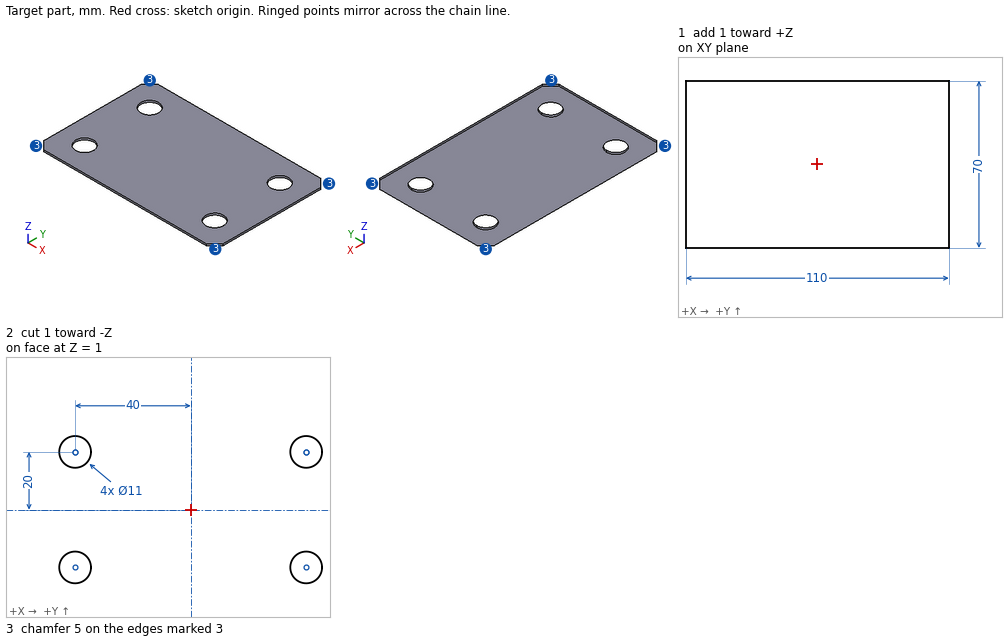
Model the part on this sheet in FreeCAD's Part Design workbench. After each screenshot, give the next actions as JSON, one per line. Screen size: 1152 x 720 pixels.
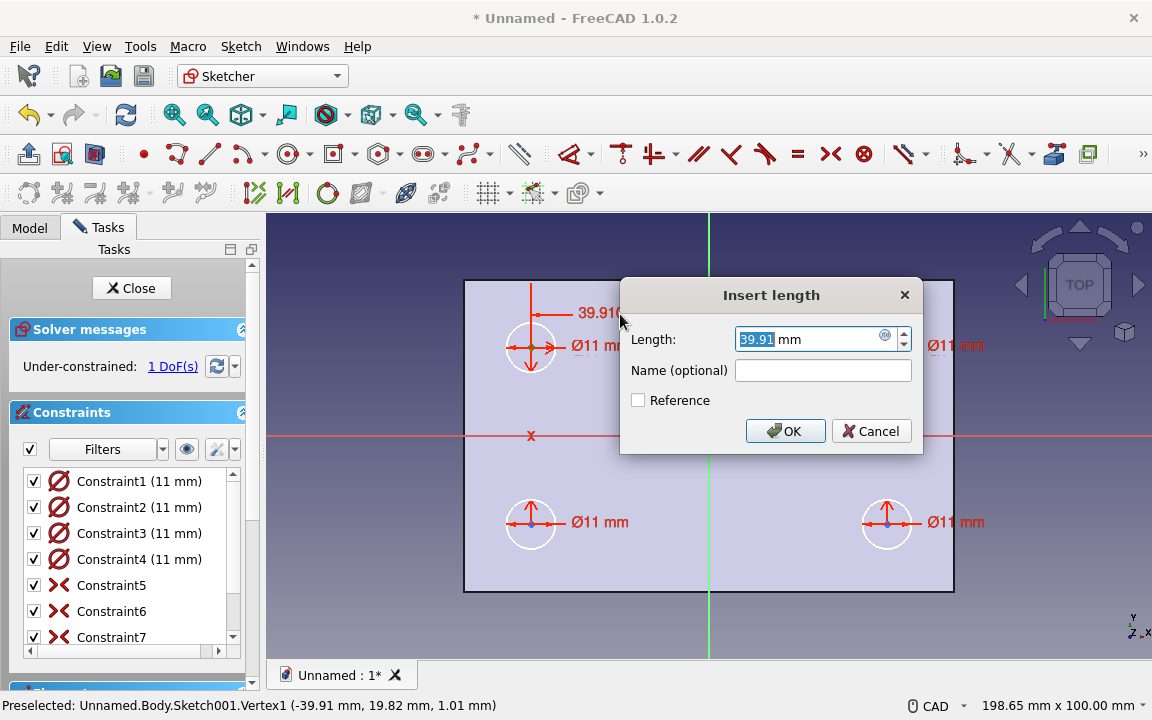
{"action": "type", "text": "40"}
{"action": "key", "text": "Return"}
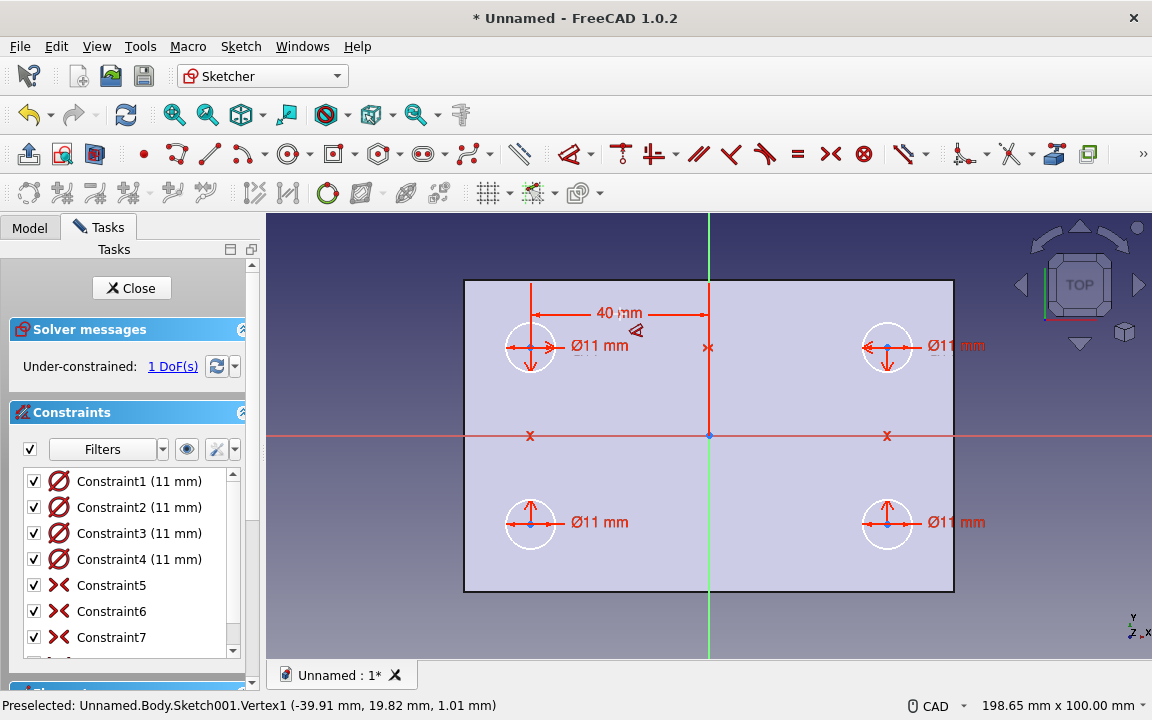
{"action": "left_click", "coordinate": [531, 348]}
{"action": "left_click", "coordinate": [497, 392]}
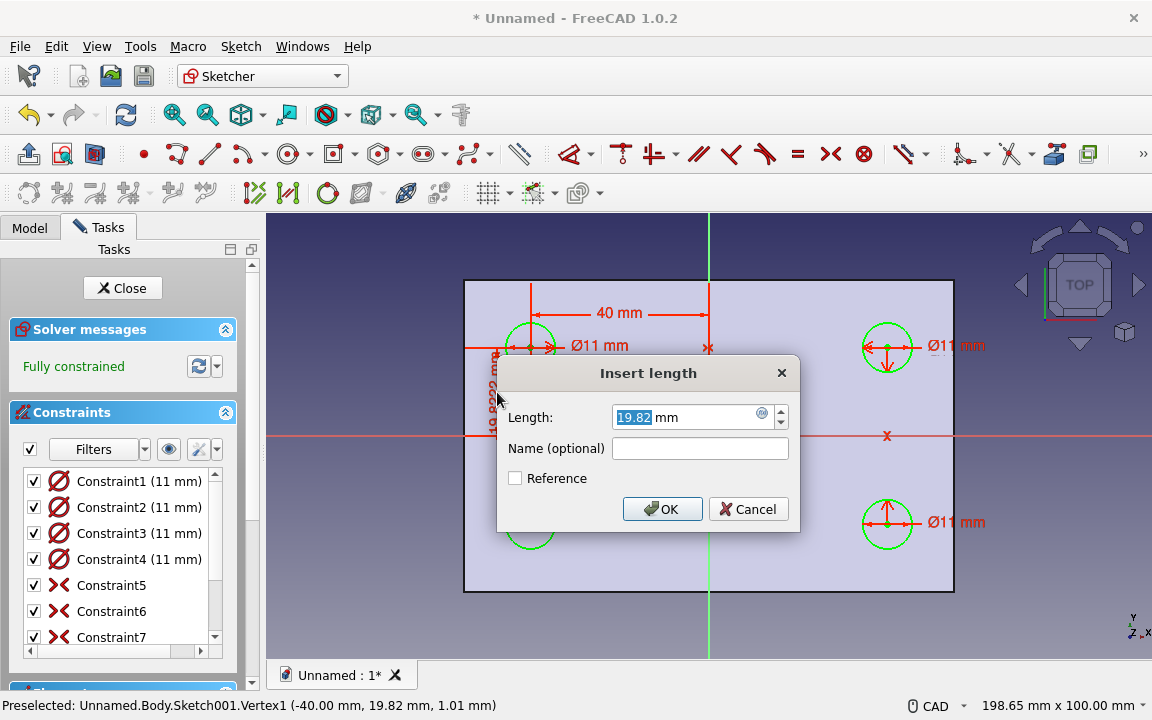
{"action": "type", "text": "20"}
{"action": "key", "text": "Return"}
{"action": "key", "text": "Escape"}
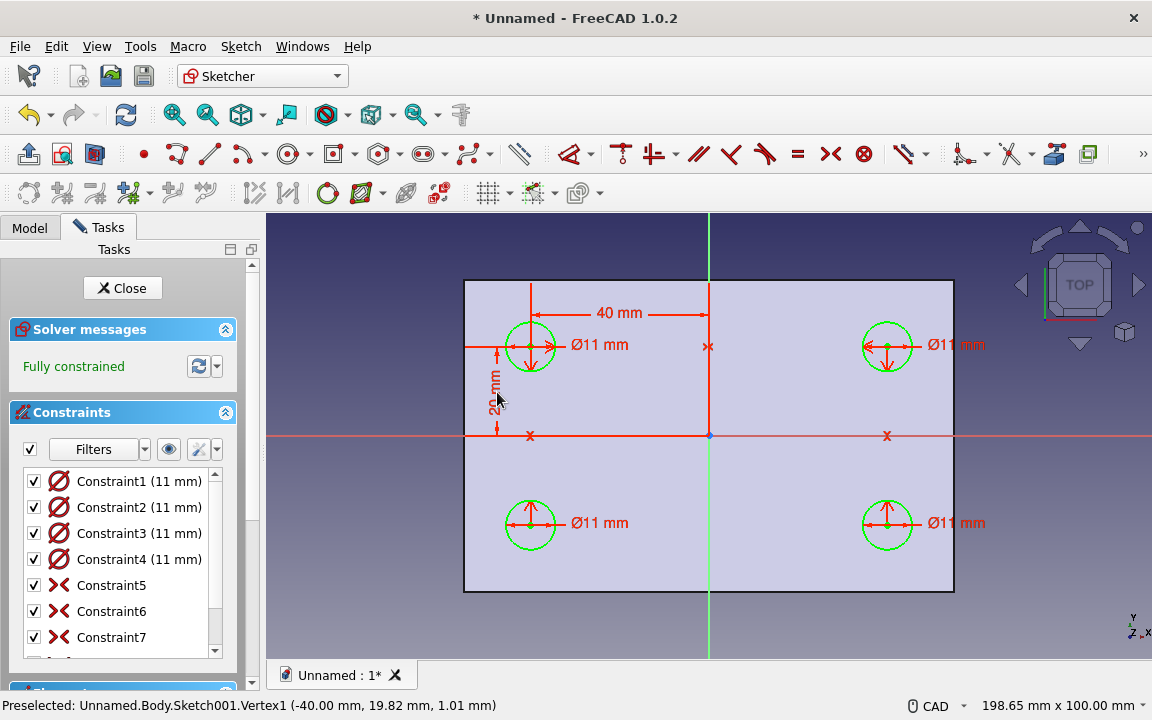
{"action": "left_click", "coordinate": [123, 288]}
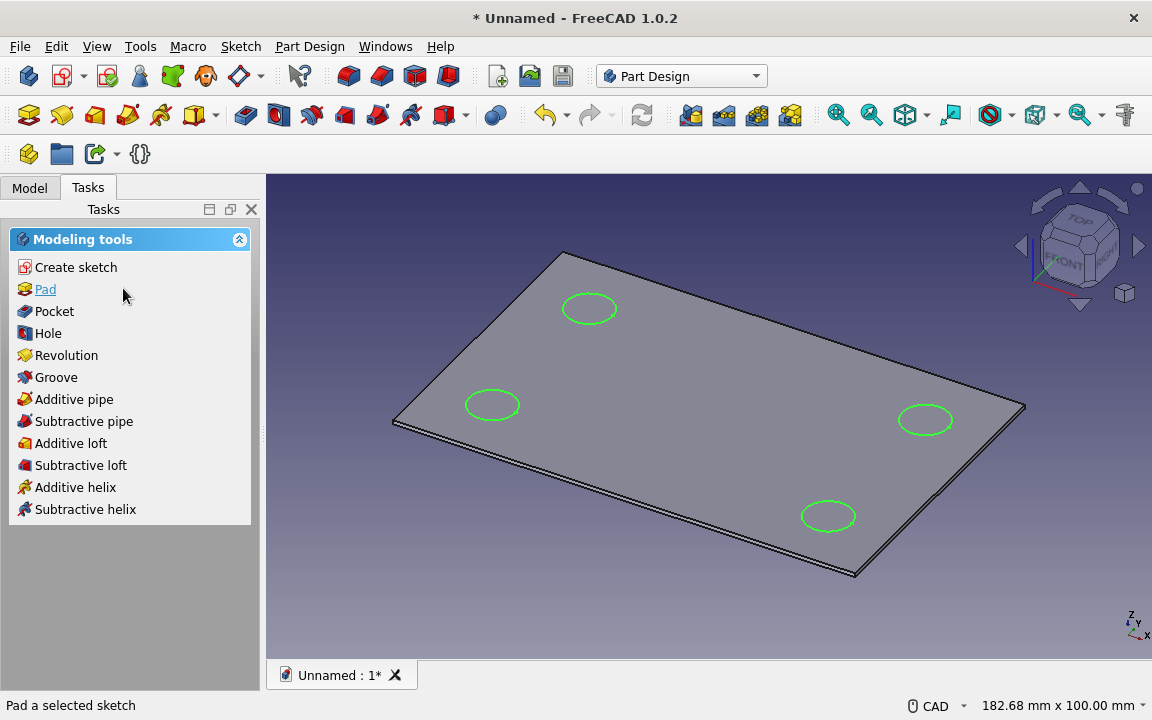
{"action": "left_click", "coordinate": [246, 116]}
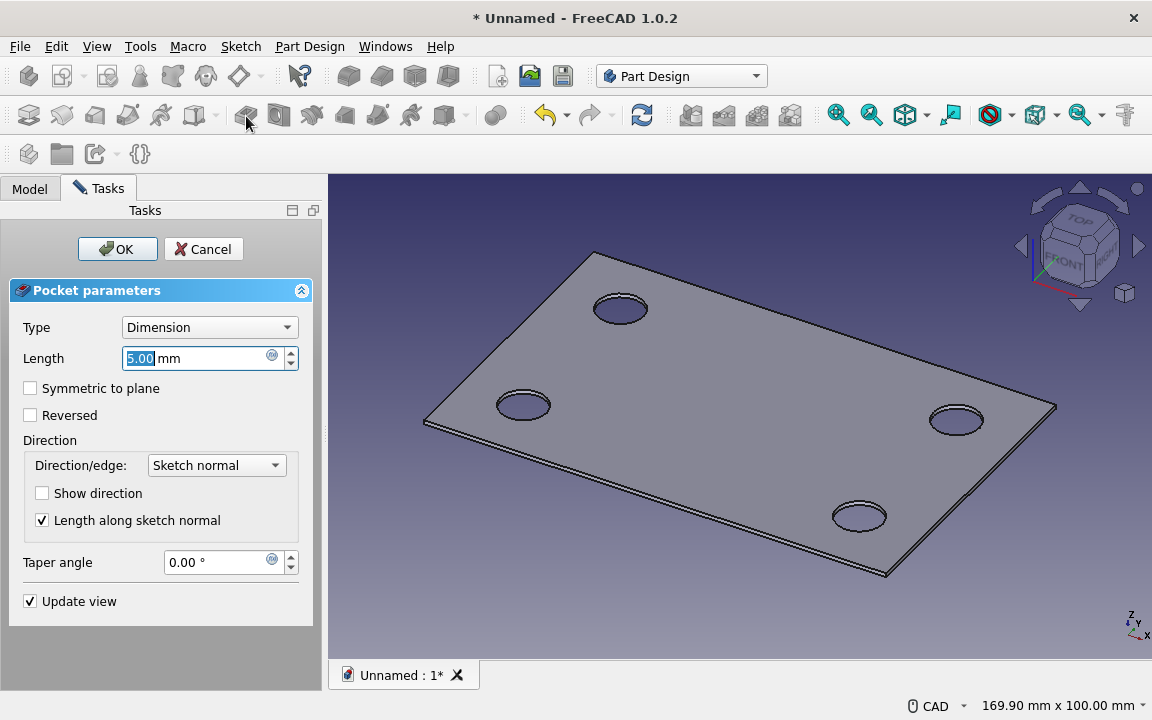
{"action": "type", "text": "1"}
{"action": "key", "text": "Tab"}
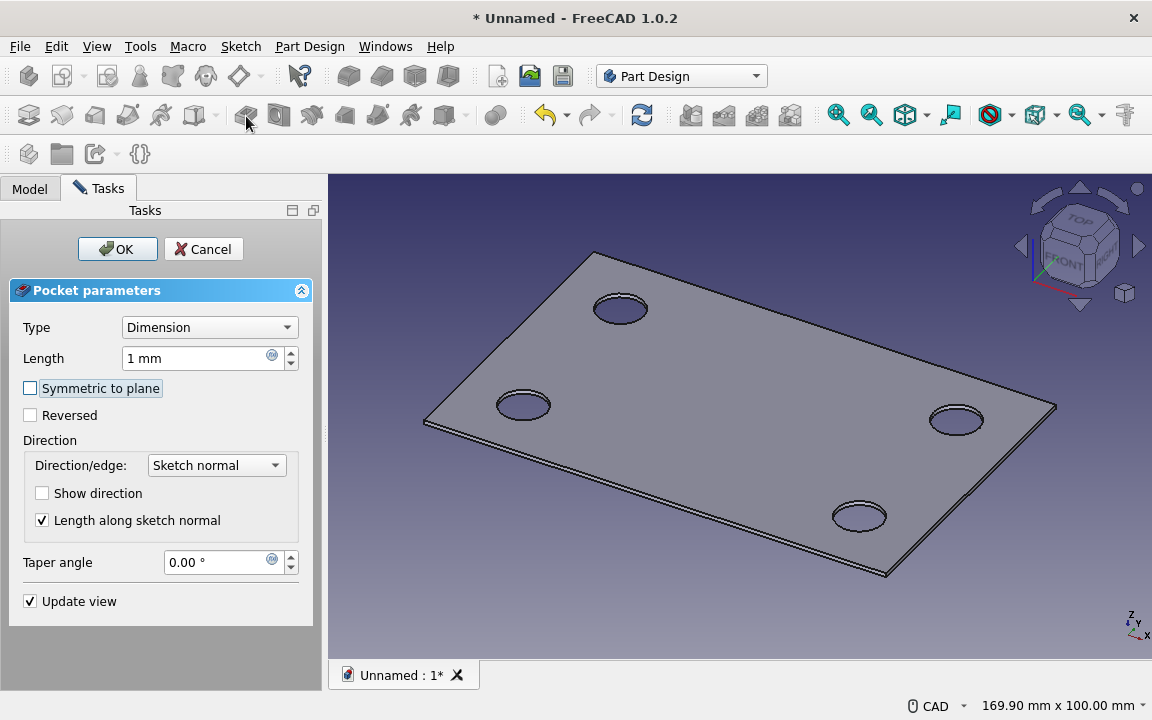
{"action": "left_click", "coordinate": [118, 249]}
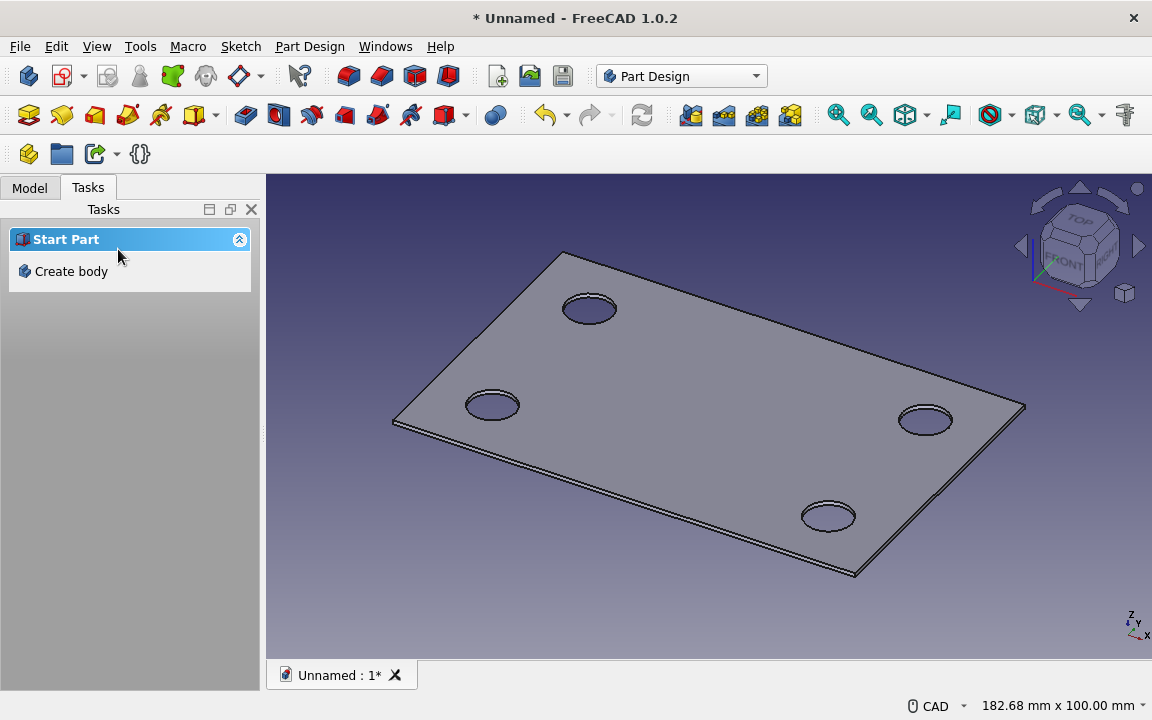
{"action": "scroll", "coordinate": [563, 253], "scroll_direction": "up", "scroll_amount": 11}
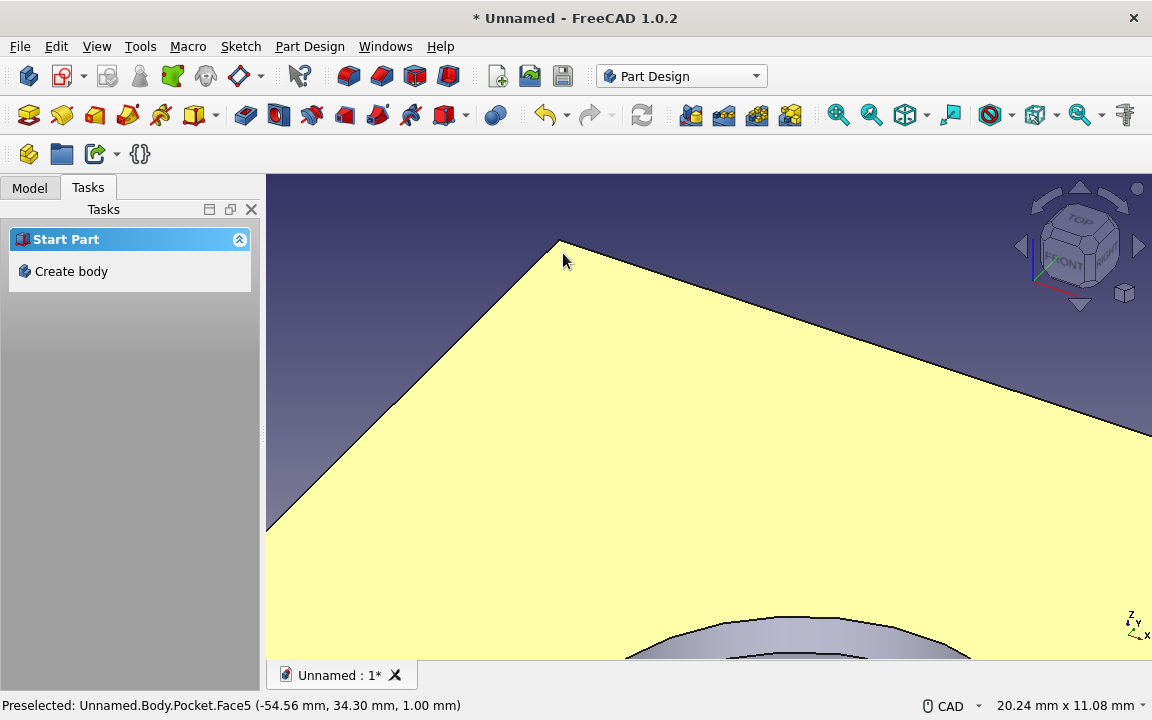
{"action": "left_click", "coordinate": [839, 116]}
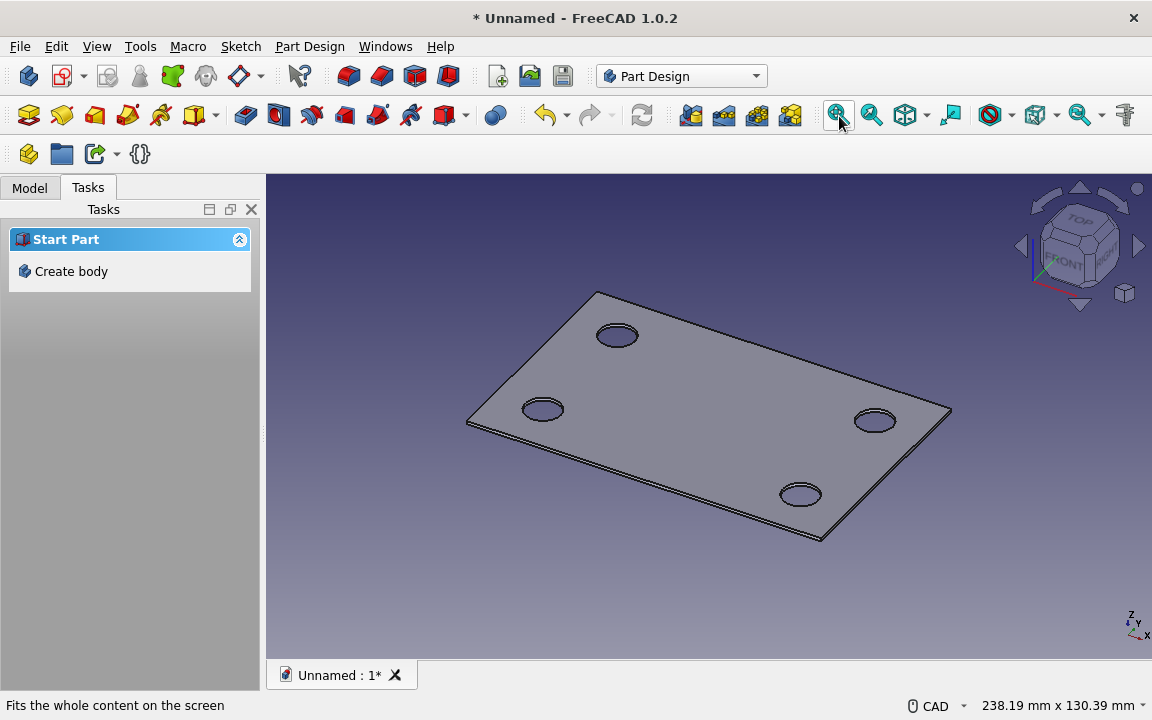
{"action": "key", "text": "0"}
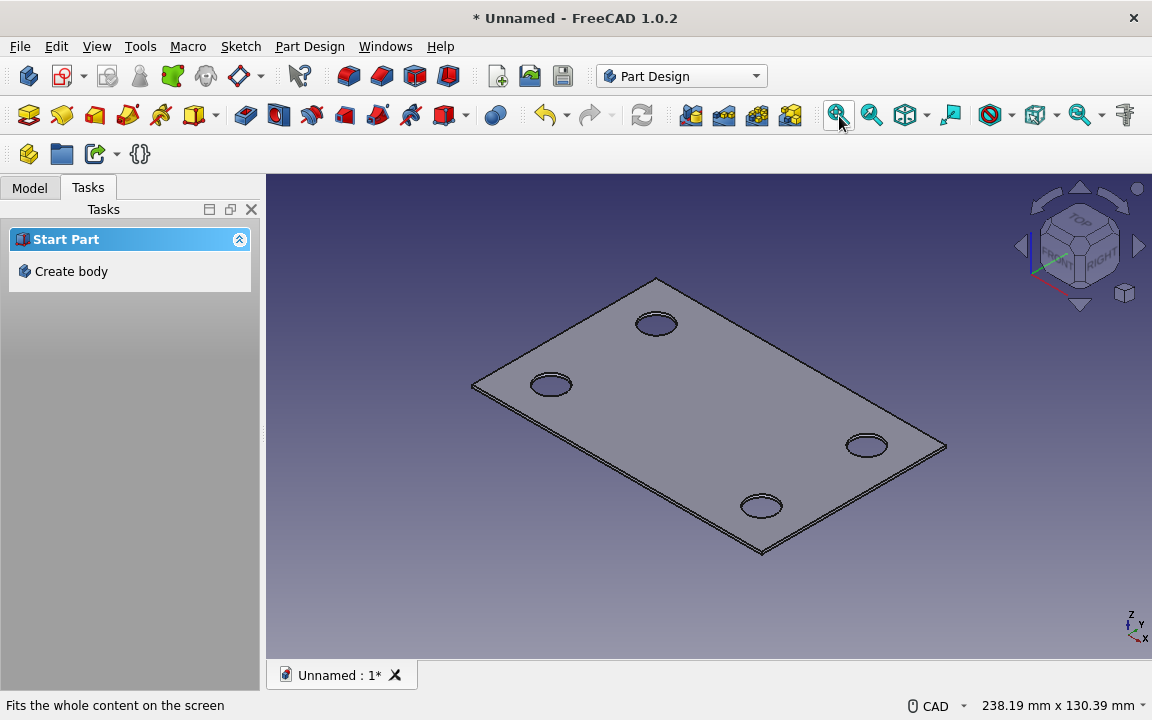
{"action": "scroll", "coordinate": [656, 279], "scroll_direction": "up", "scroll_amount": 12}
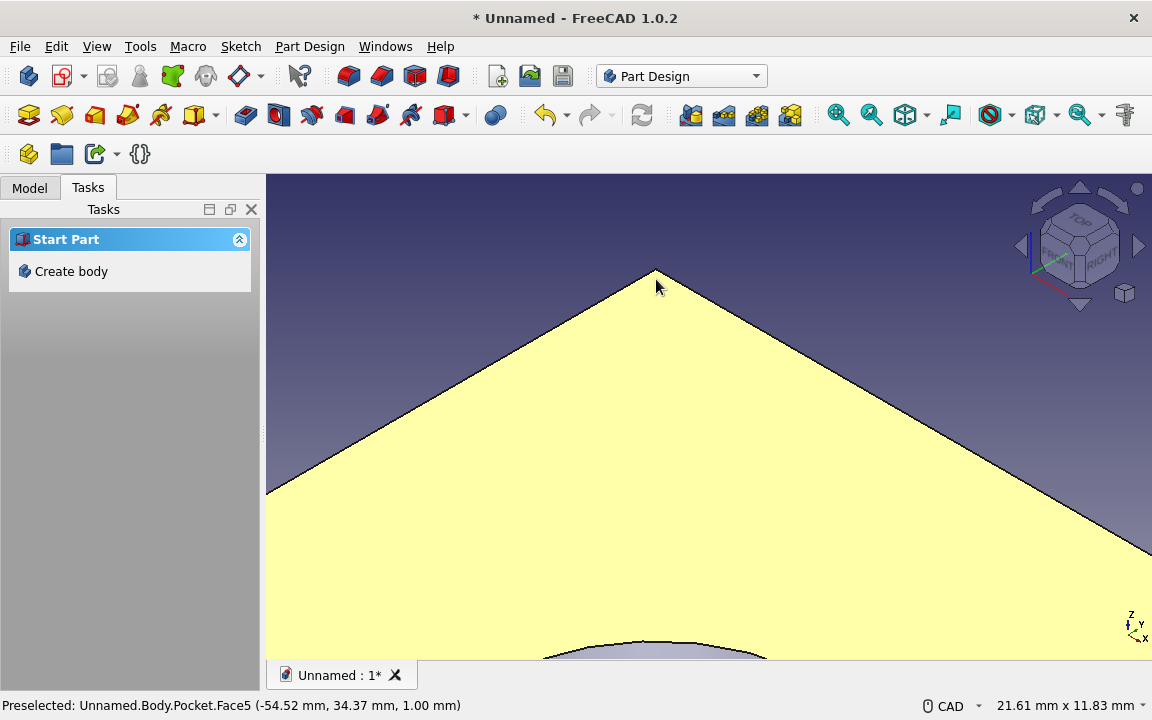
{"action": "left_click", "coordinate": [839, 116]}